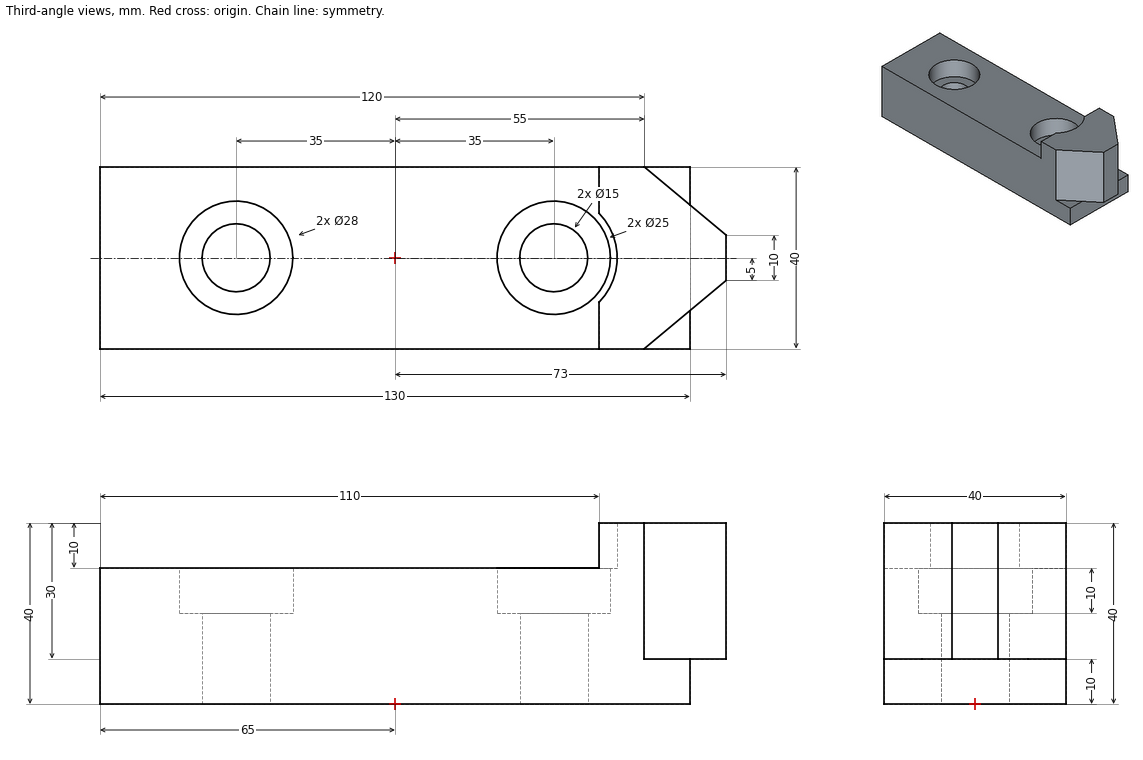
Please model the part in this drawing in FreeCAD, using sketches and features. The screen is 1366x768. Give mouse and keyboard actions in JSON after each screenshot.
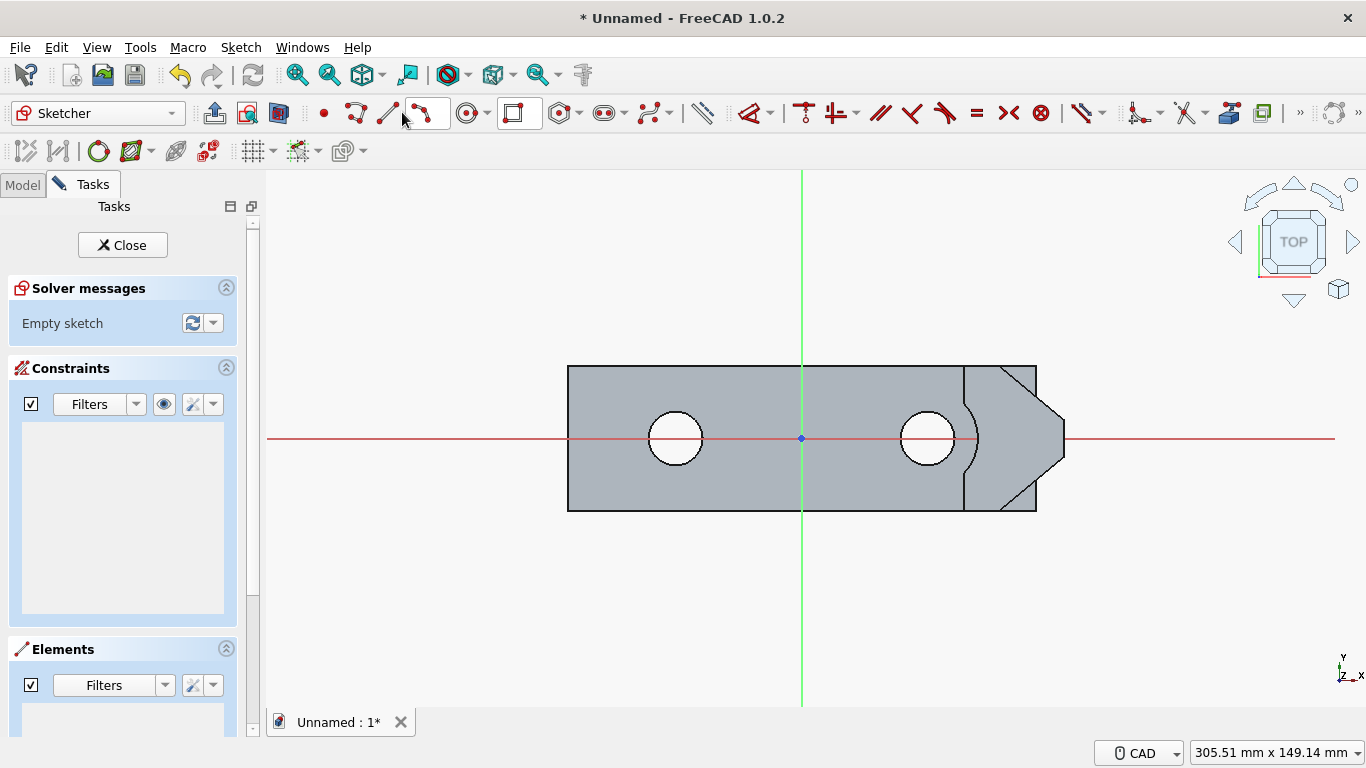
{"action": "scroll", "coordinate": [867, 438], "scroll_direction": "up", "scroll_amount": 3}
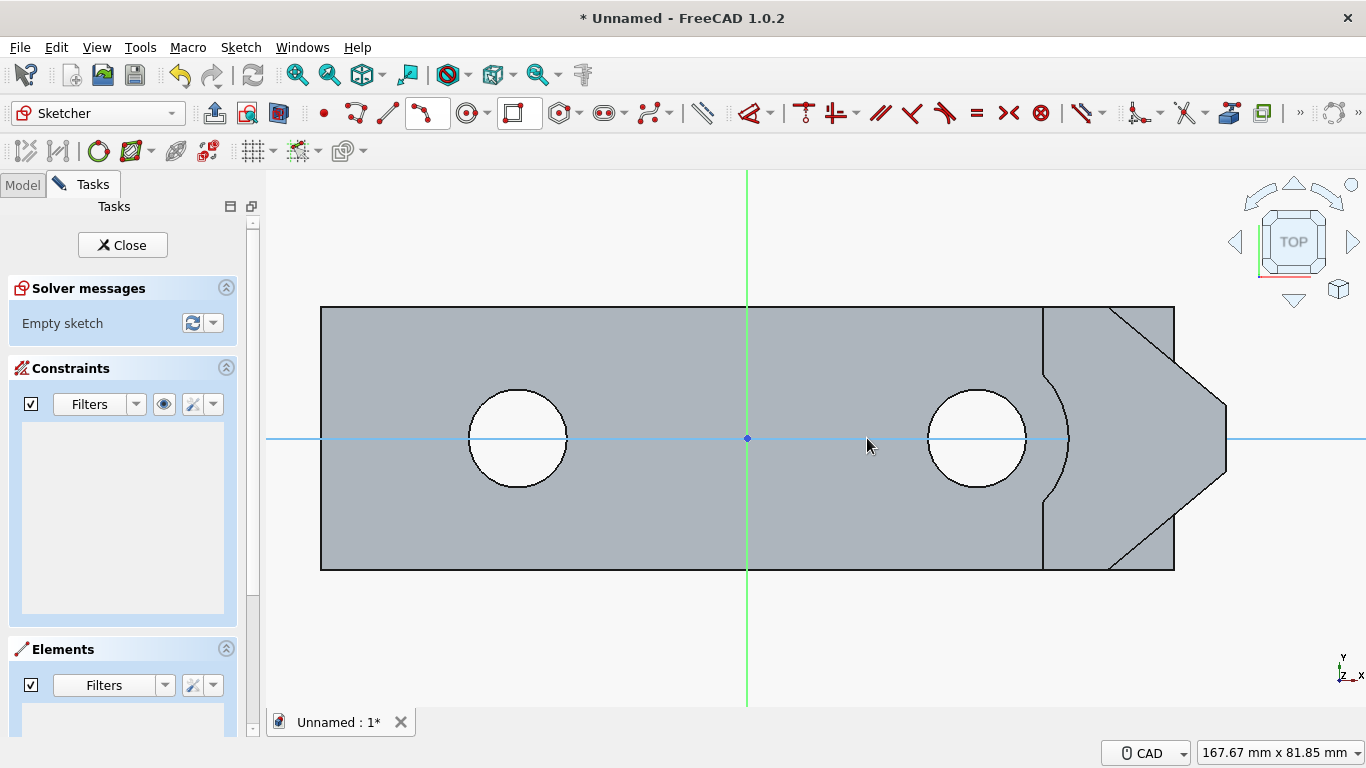
{"action": "left_click", "coordinate": [468, 114]}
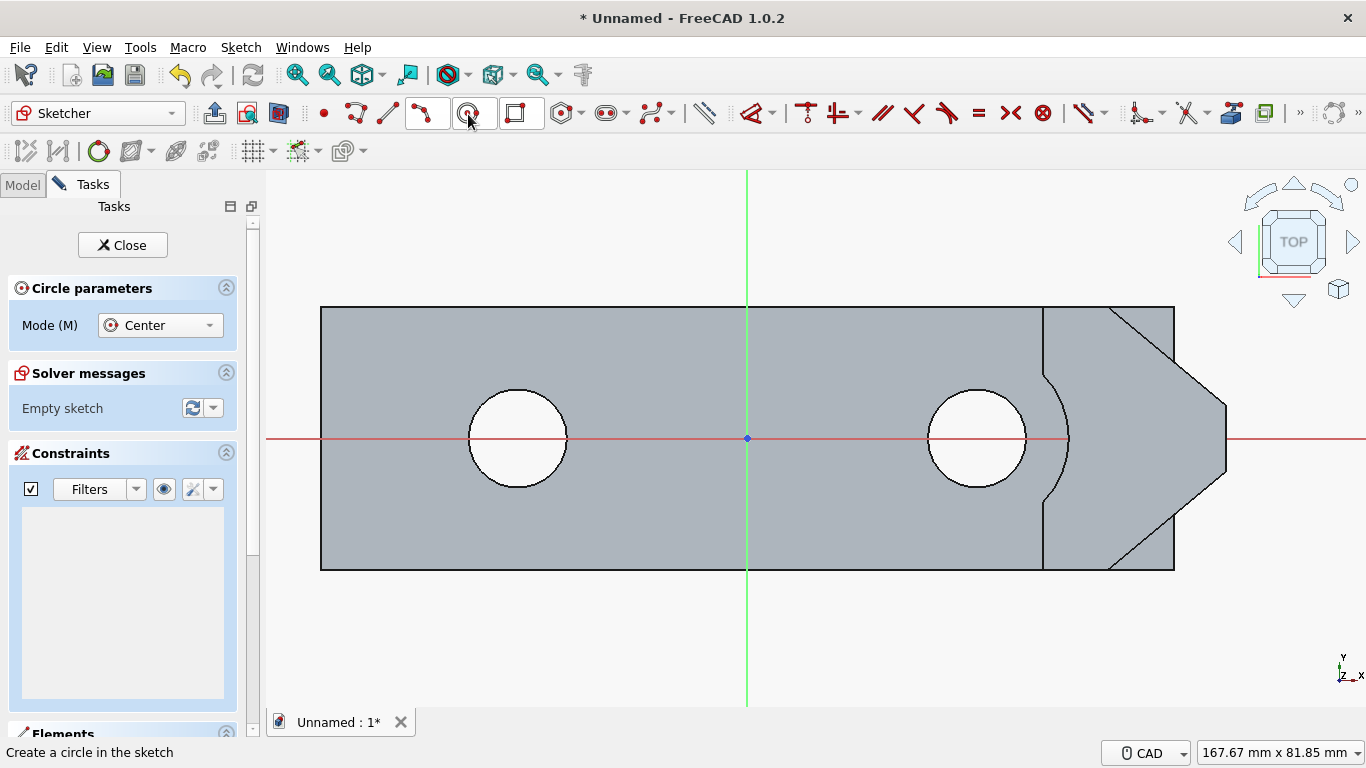
{"action": "left_click", "coordinate": [977, 438]}
{"action": "left_click", "coordinate": [1035, 381]}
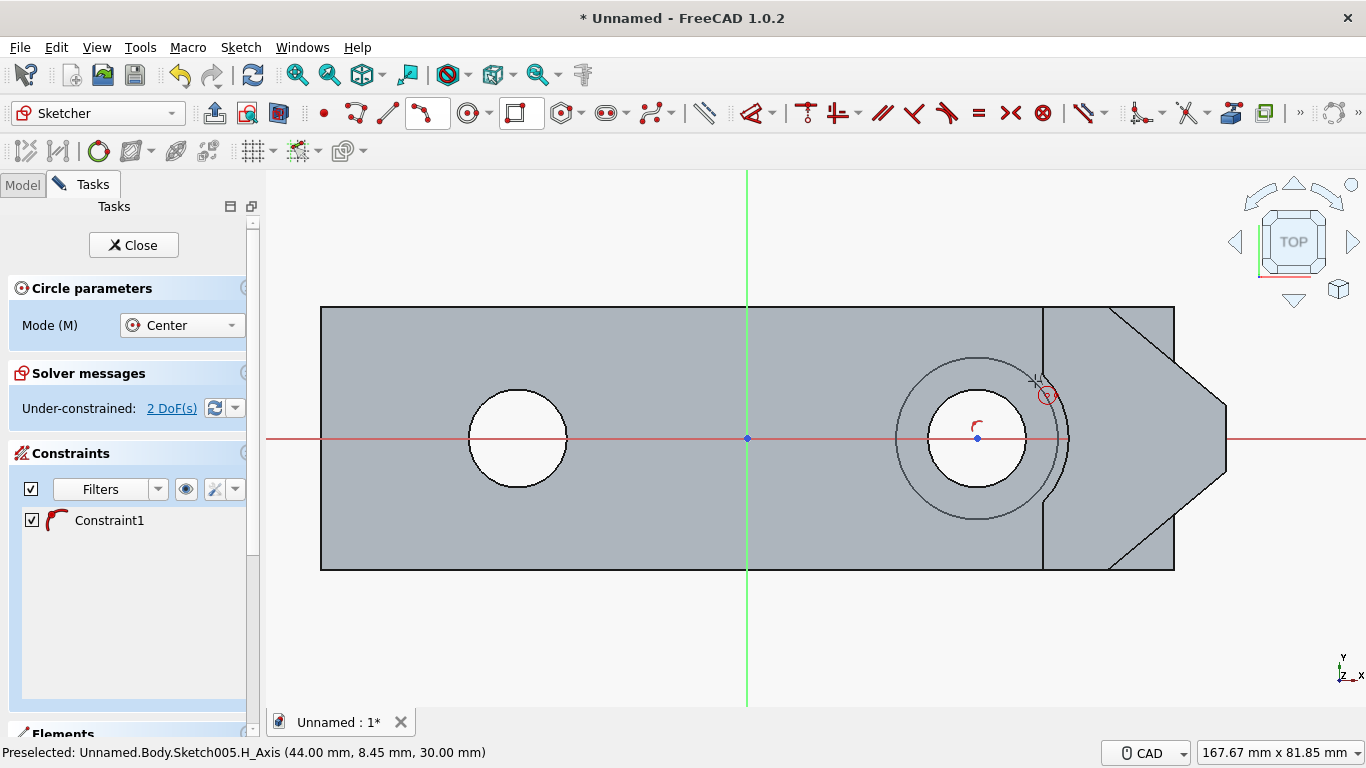
{"action": "left_click", "coordinate": [518, 438]}
{"action": "left_click", "coordinate": [576, 381]}
{"action": "key", "text": "Escape"}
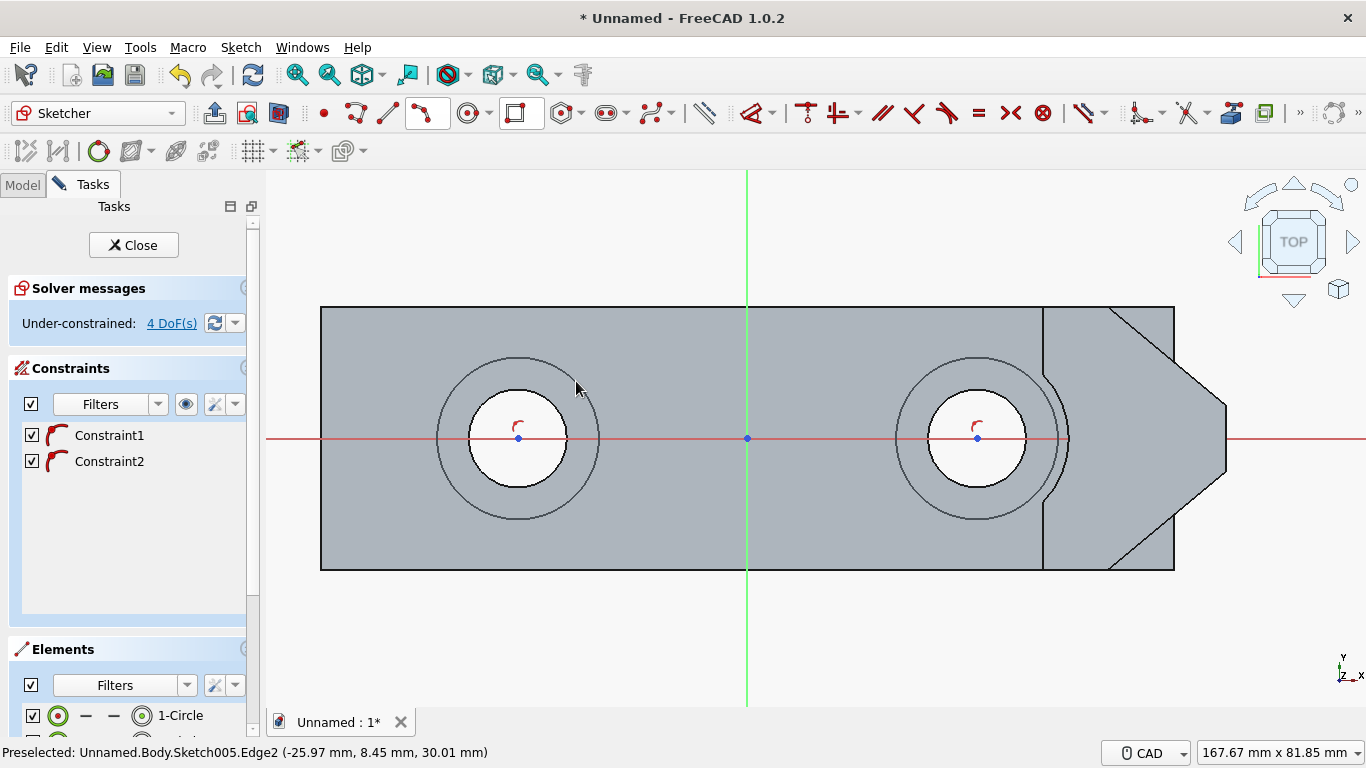
{"action": "left_click", "coordinate": [1034, 381]}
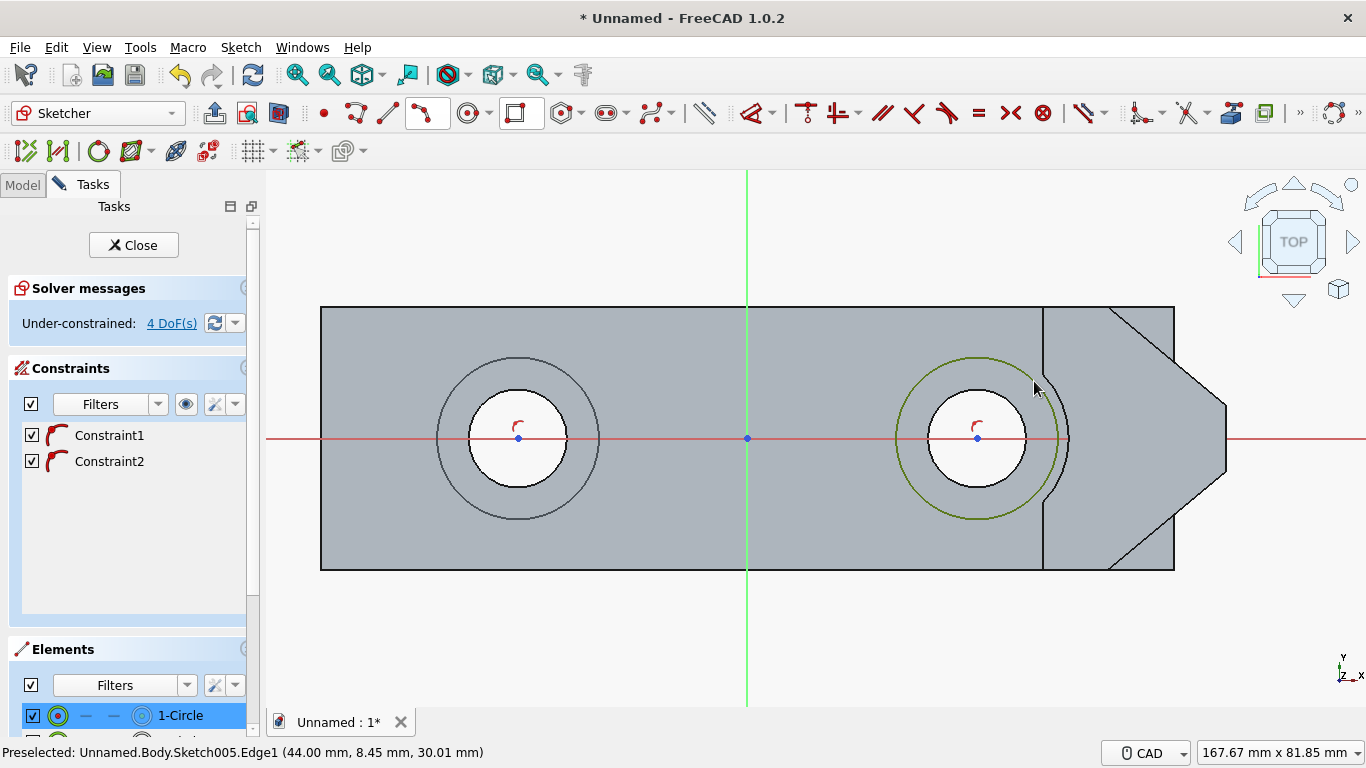
{"action": "left_click", "coordinate": [575, 381]}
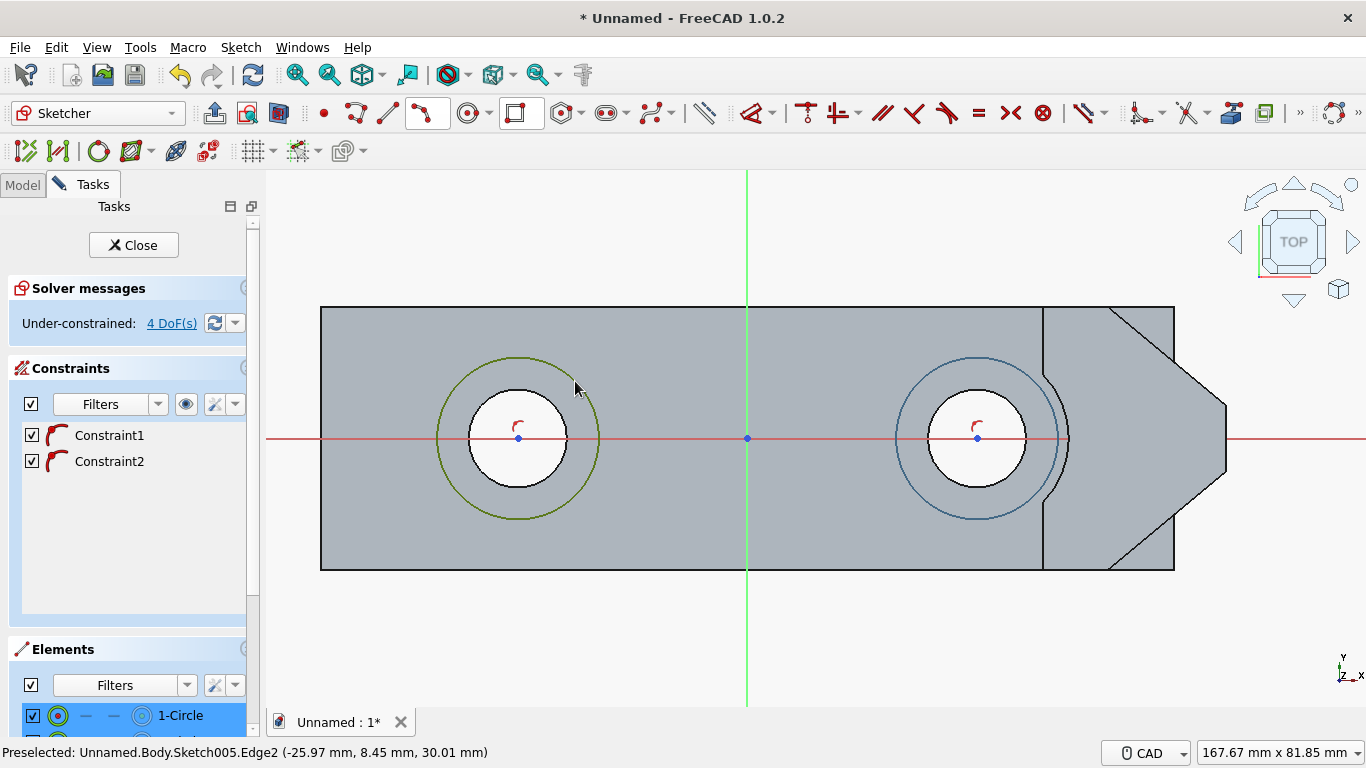
{"action": "left_click", "coordinate": [980, 114]}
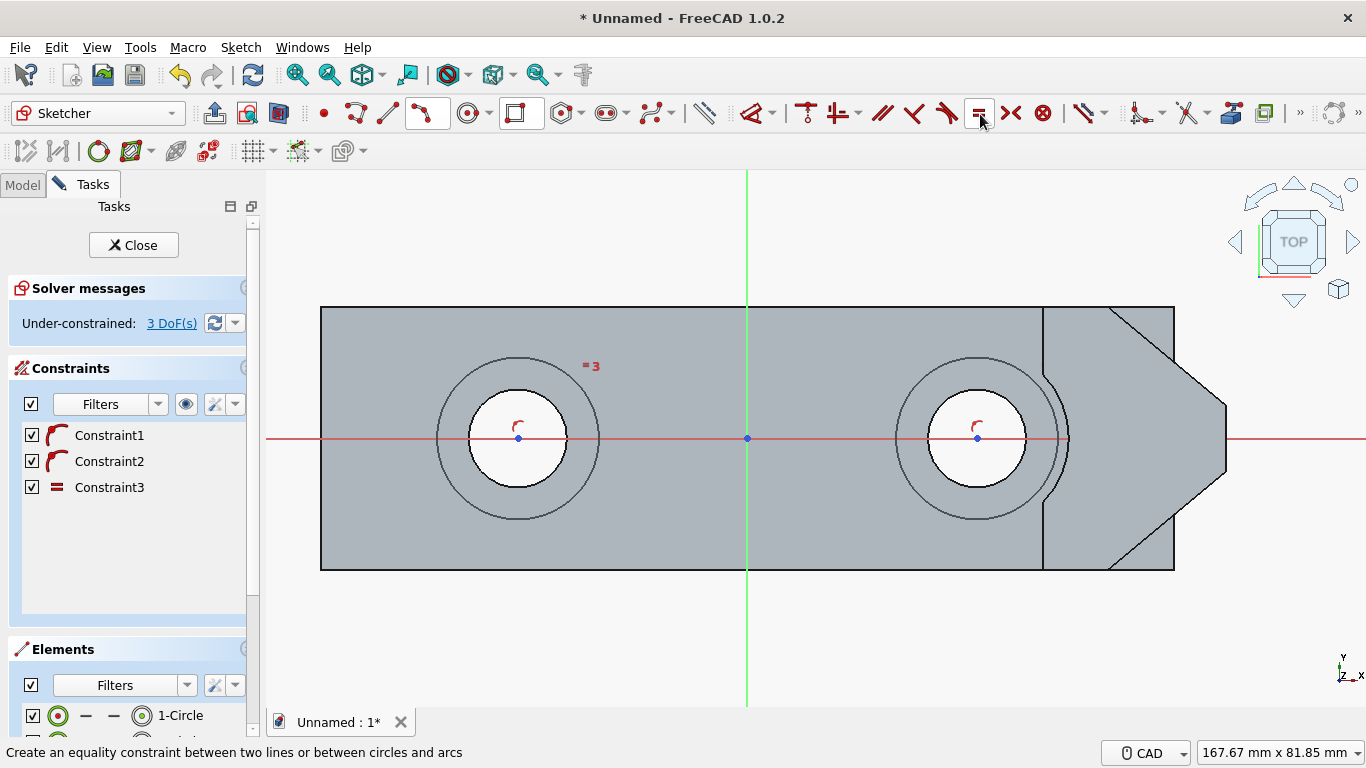
{"action": "left_click", "coordinate": [752, 114]}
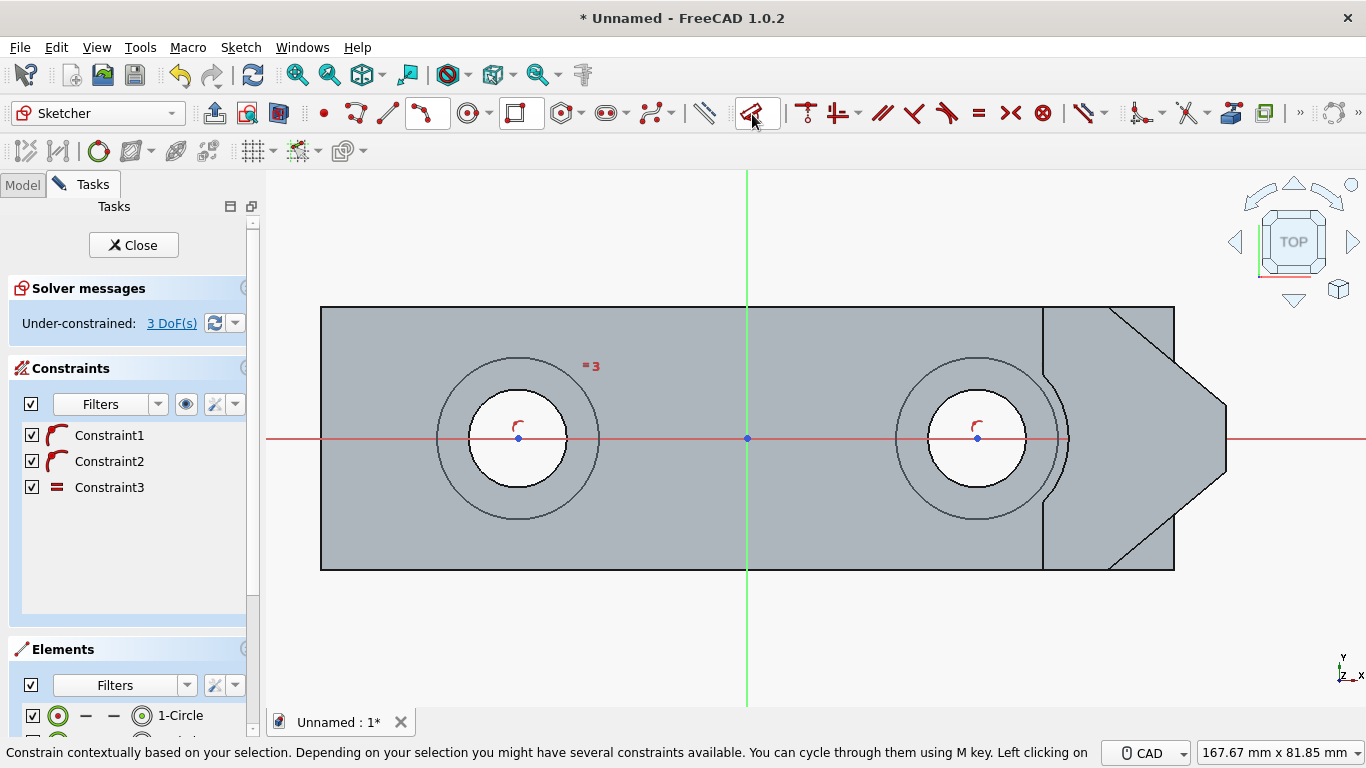
{"action": "left_click", "coordinate": [1034, 381]}
{"action": "left_click", "coordinate": [1057, 358]}